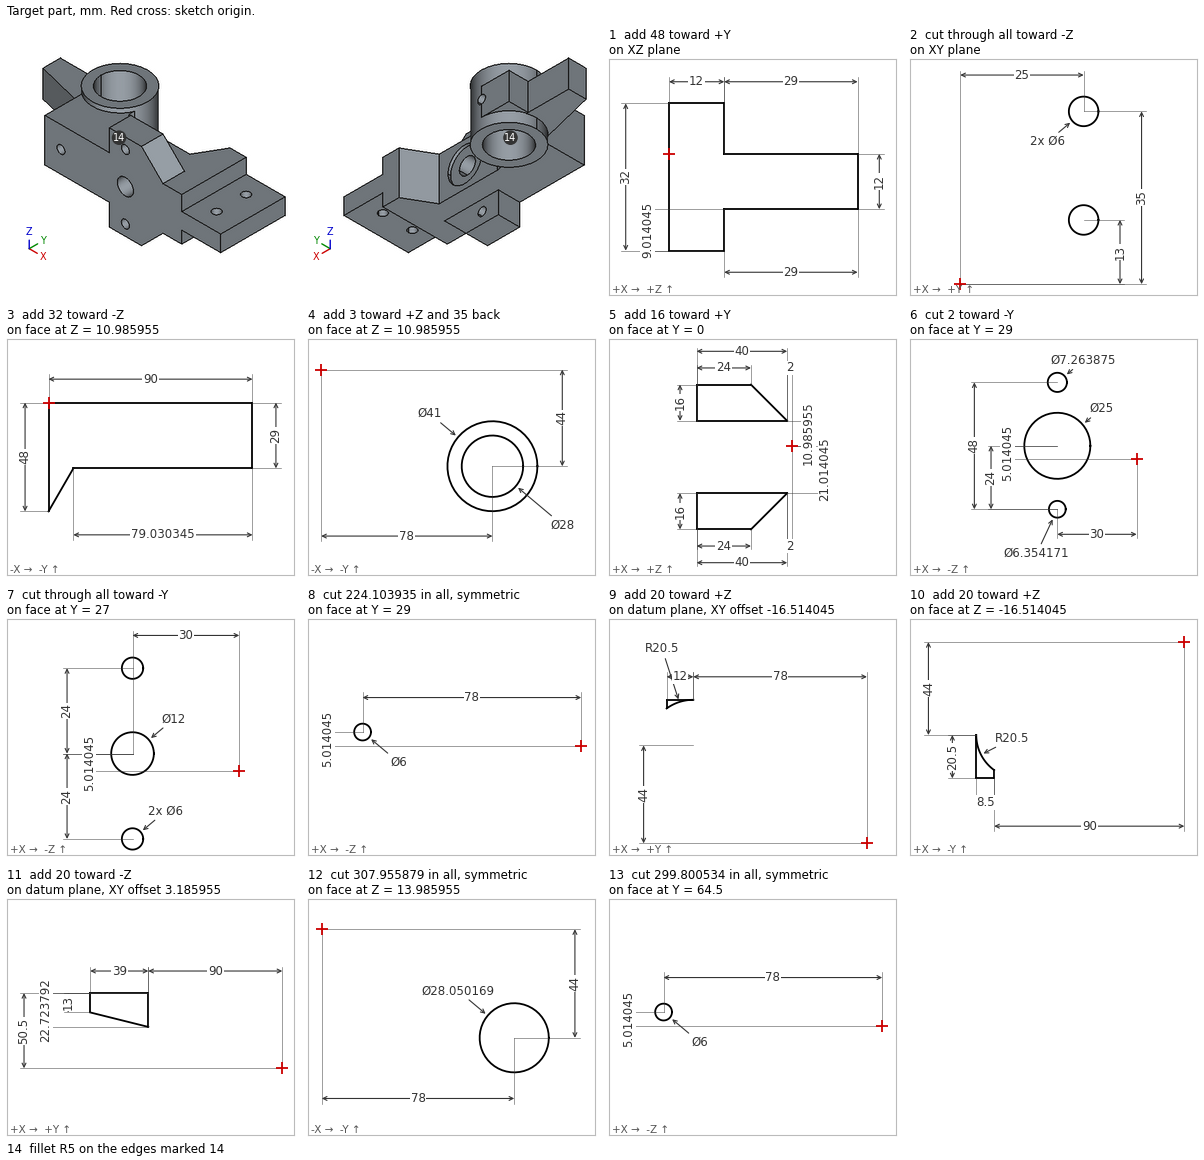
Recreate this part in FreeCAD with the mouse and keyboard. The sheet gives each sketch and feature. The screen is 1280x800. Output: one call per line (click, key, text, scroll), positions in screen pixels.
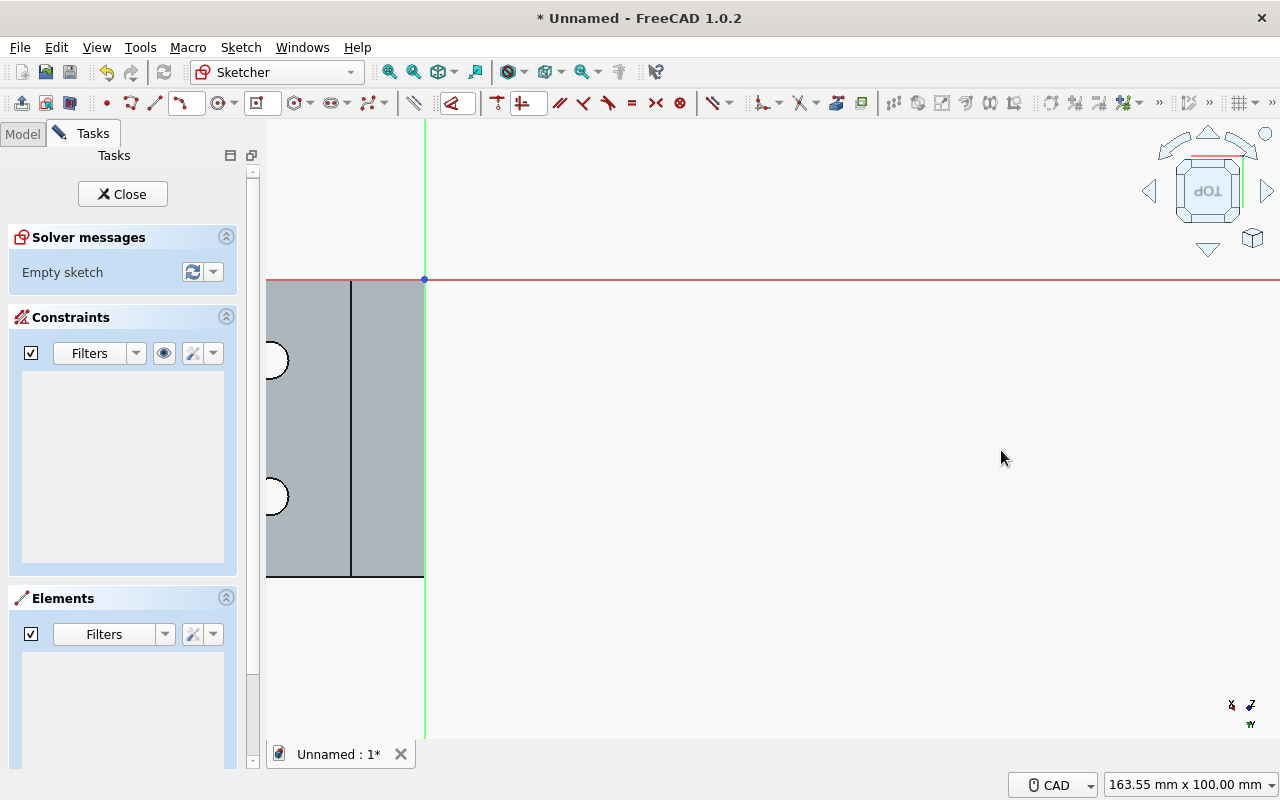
key(g)
key(m)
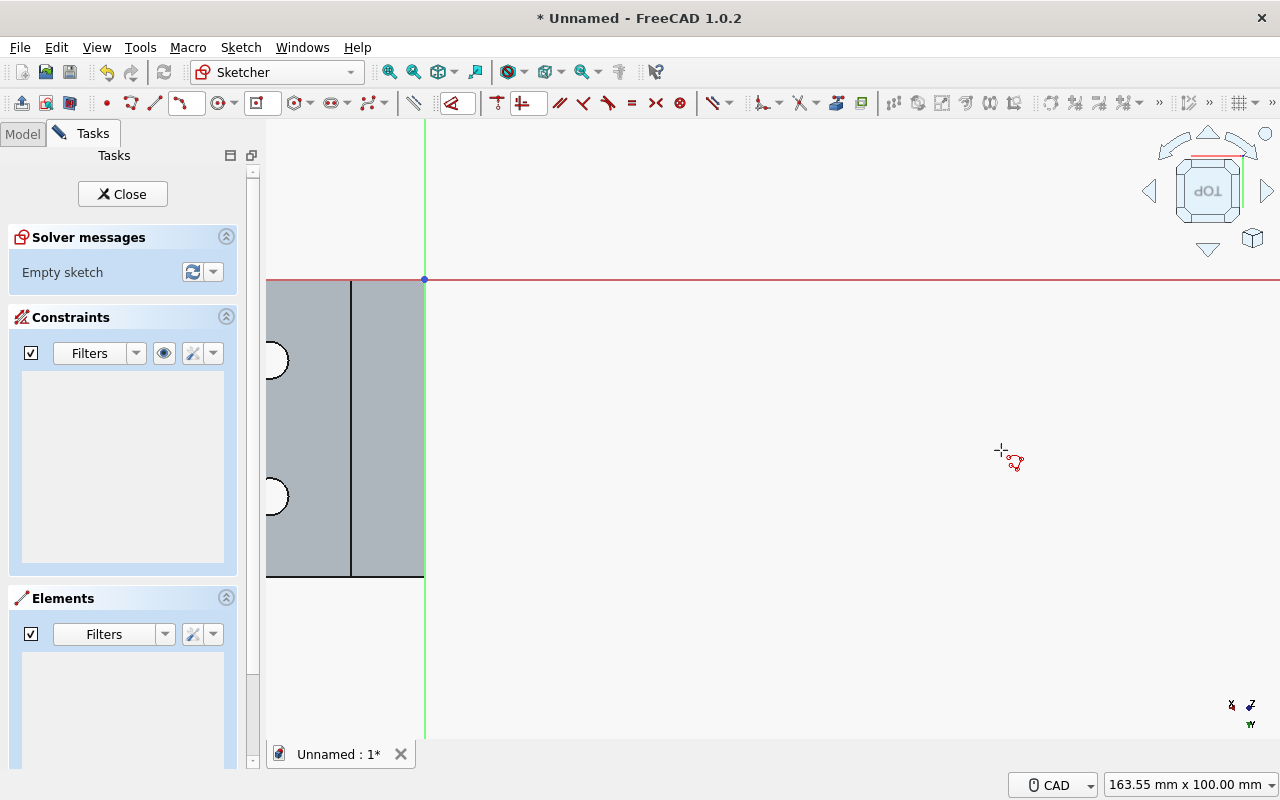
click(425, 280)
click(434, 577)
click(493, 460)
click(983, 460)
click(983, 289)
click(425, 280)
key(Escape)
key(Escape)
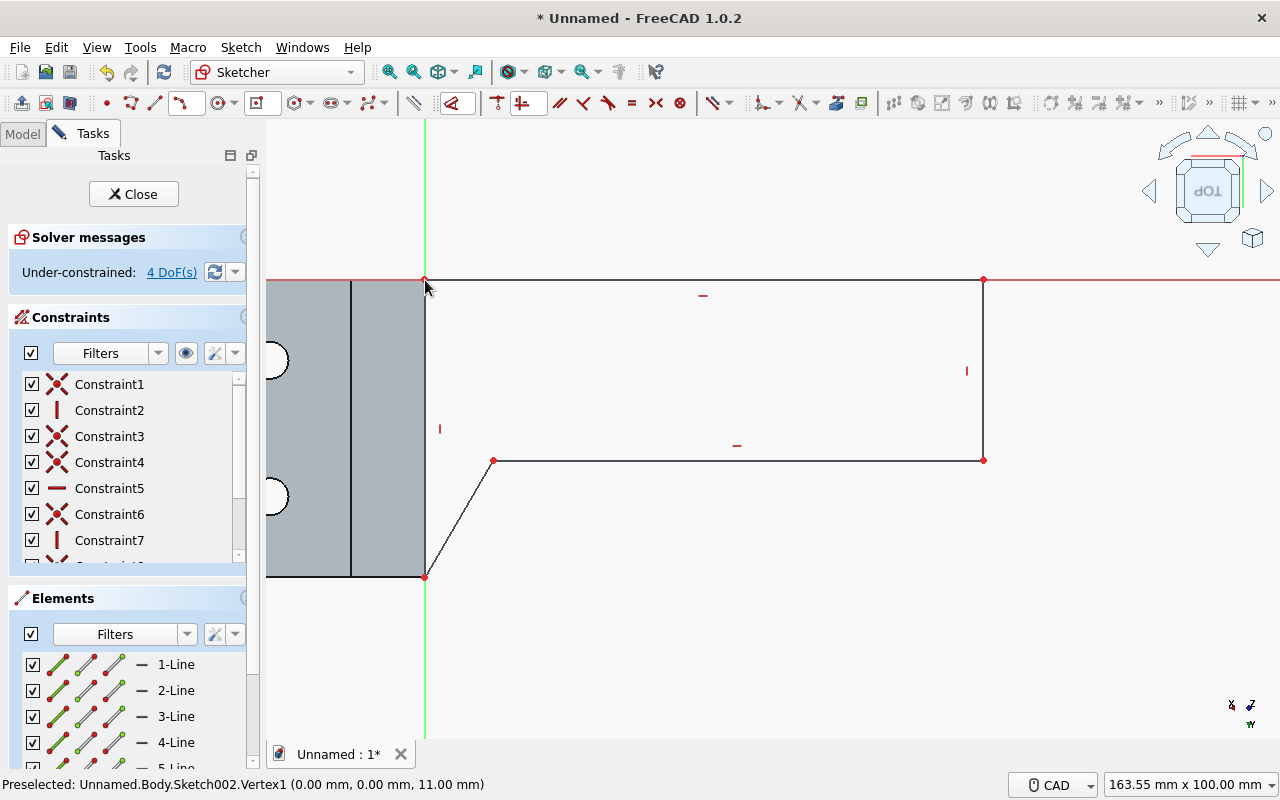
click(425, 369)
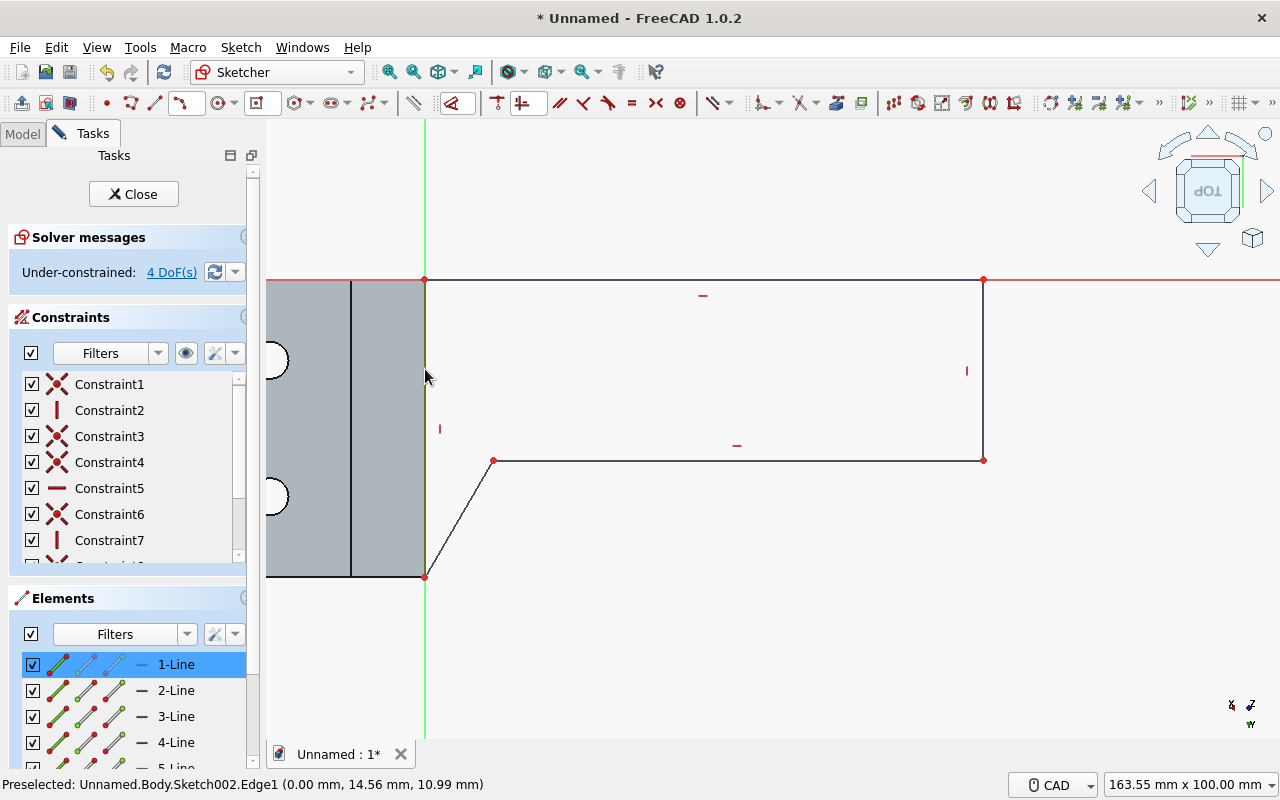
key(i)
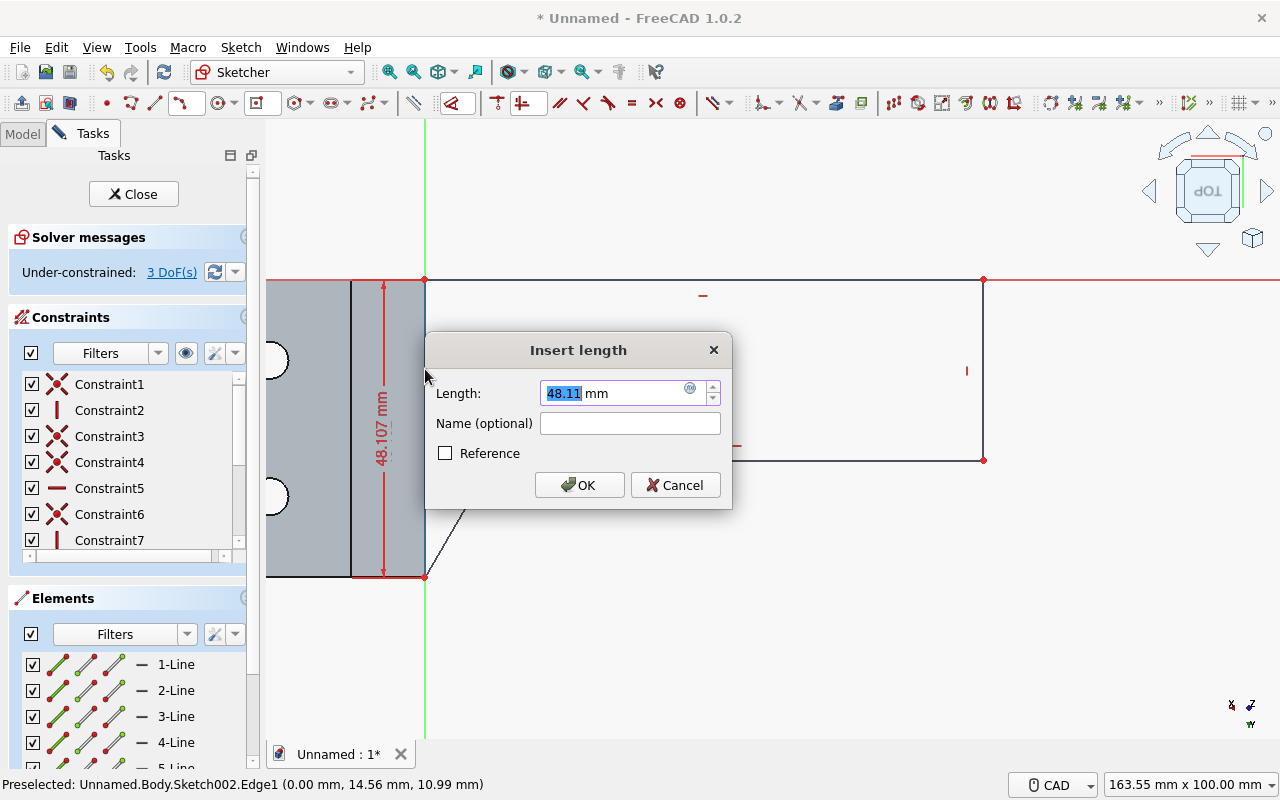
text(48)
key(Return)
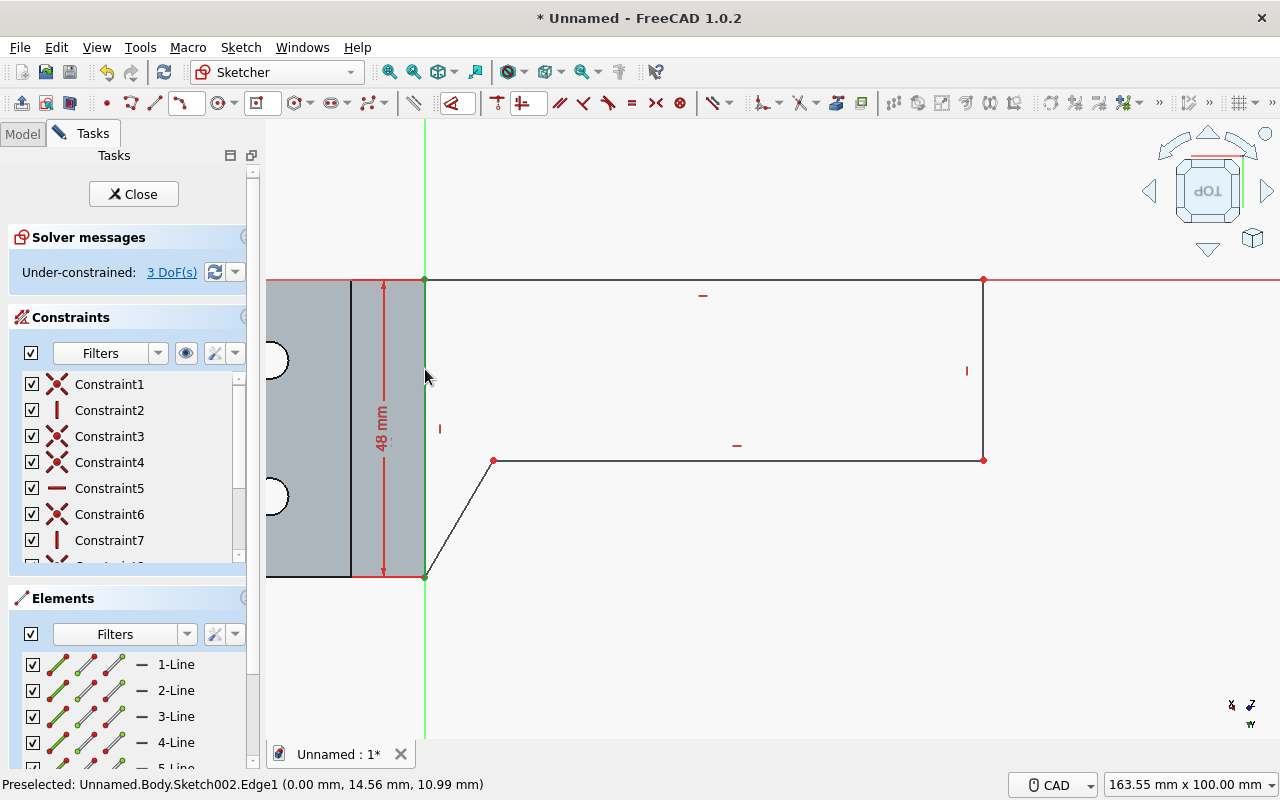
click(983, 407)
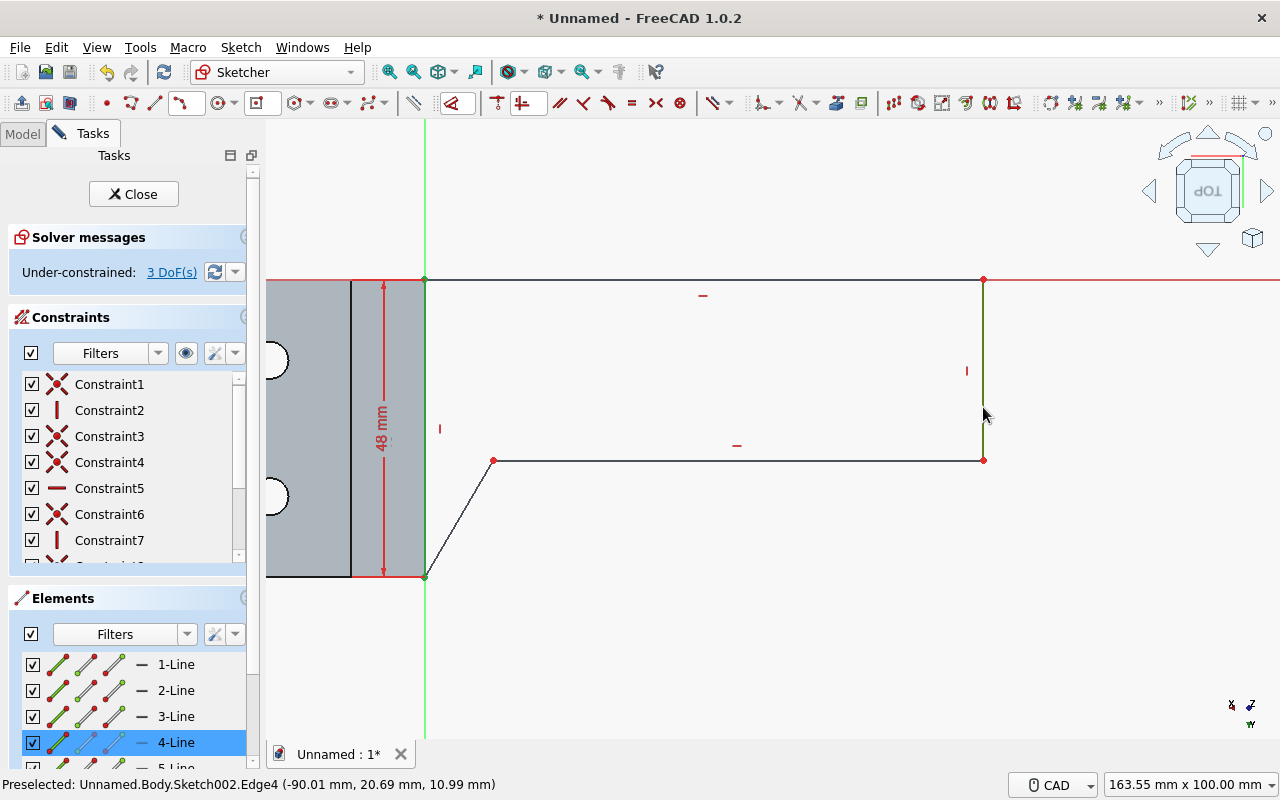
key(i)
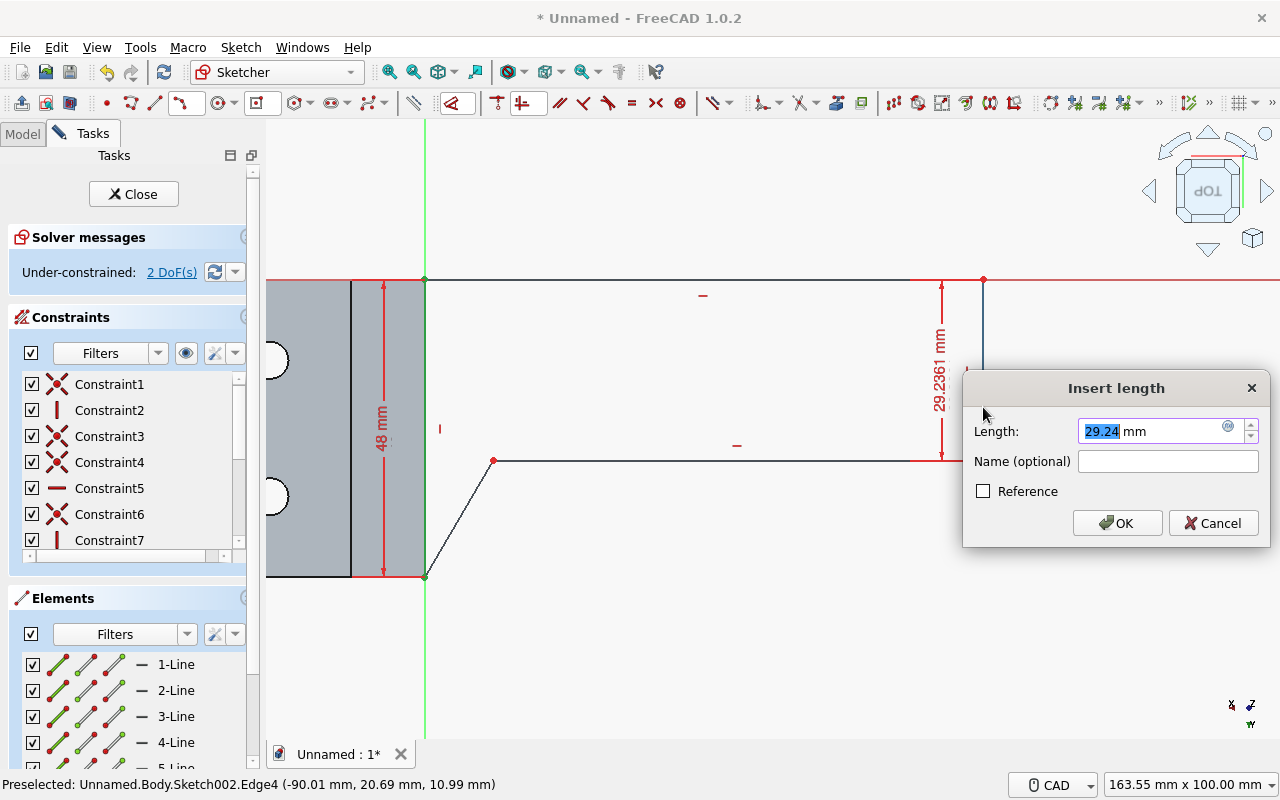
text(29)
key(Return)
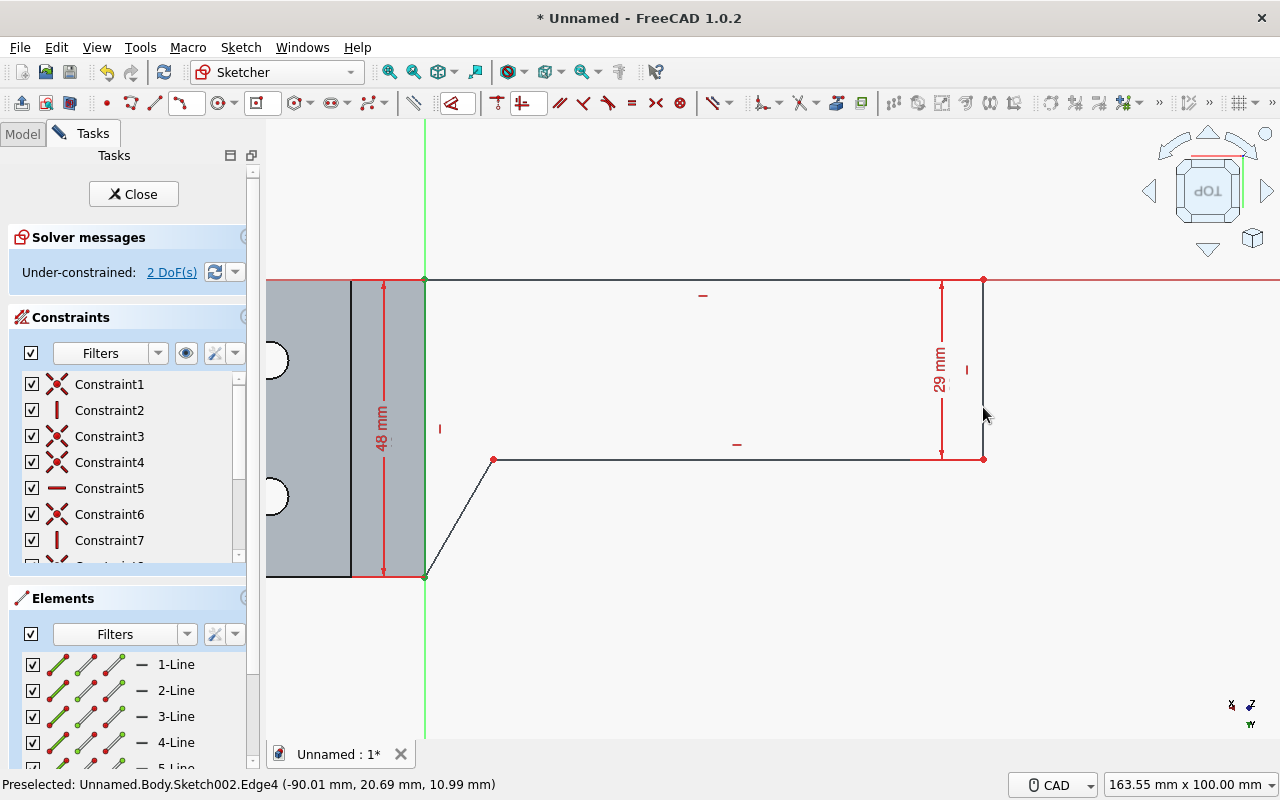
click(816, 280)